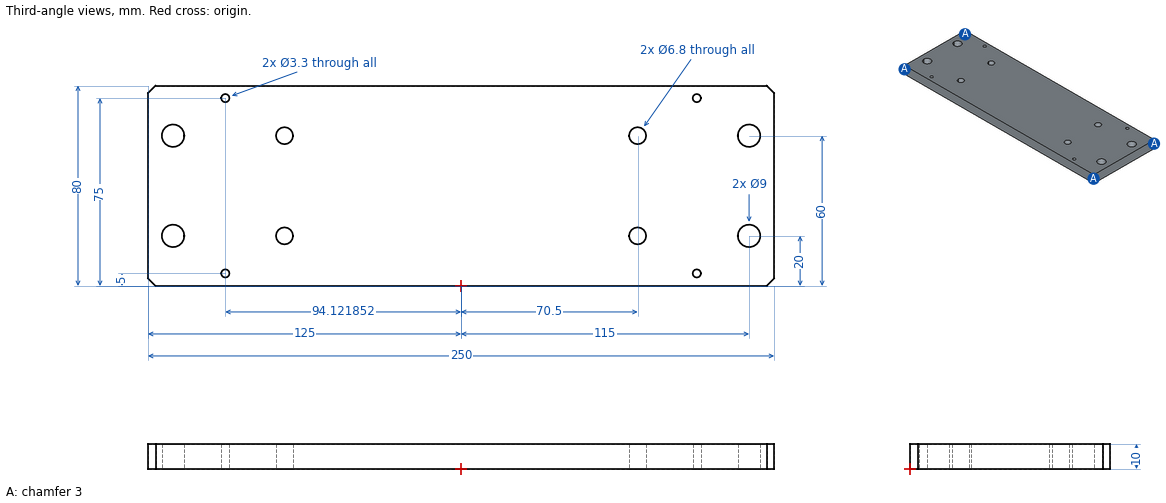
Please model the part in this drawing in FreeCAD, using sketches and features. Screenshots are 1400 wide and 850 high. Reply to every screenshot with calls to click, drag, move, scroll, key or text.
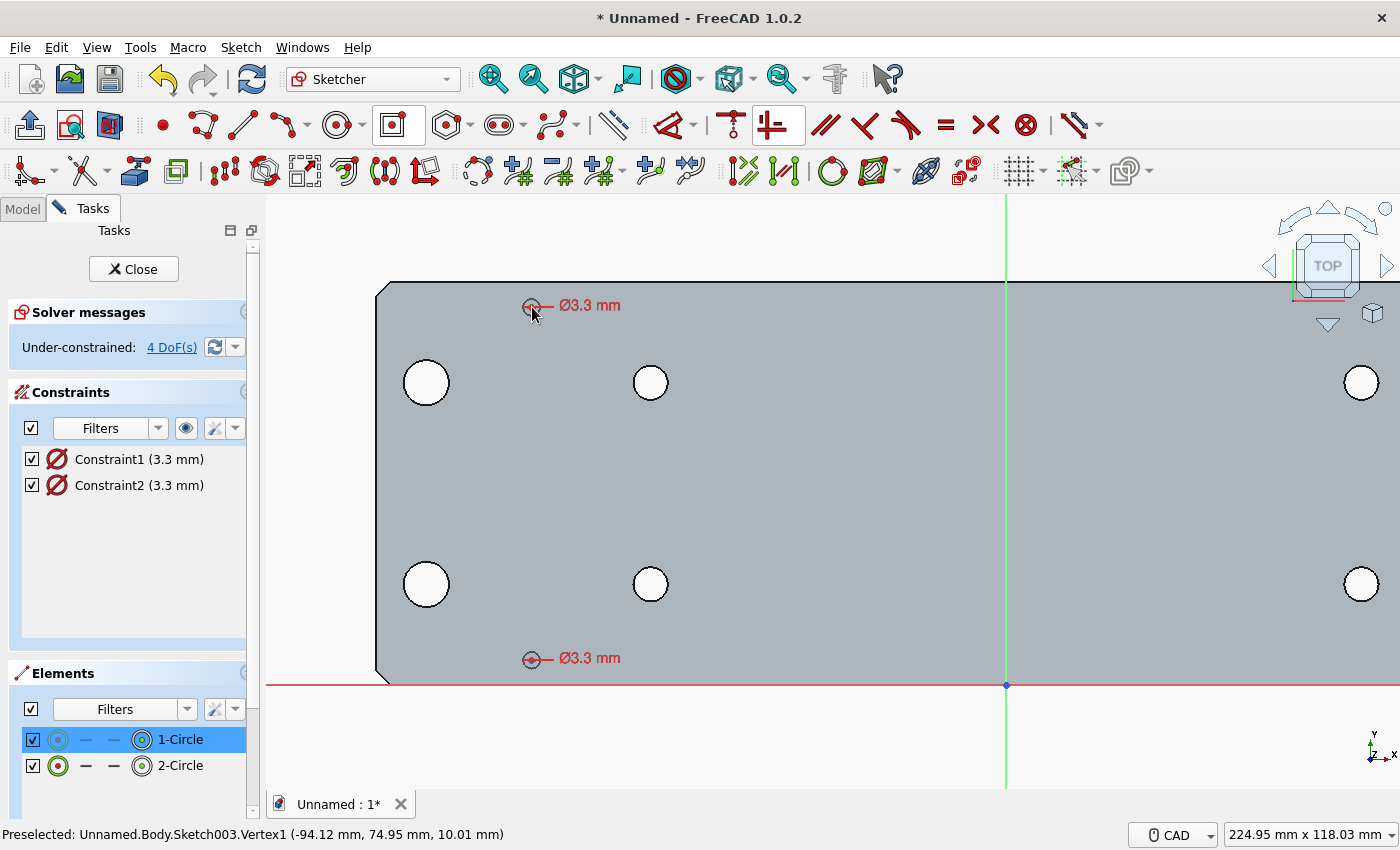
click(532, 660)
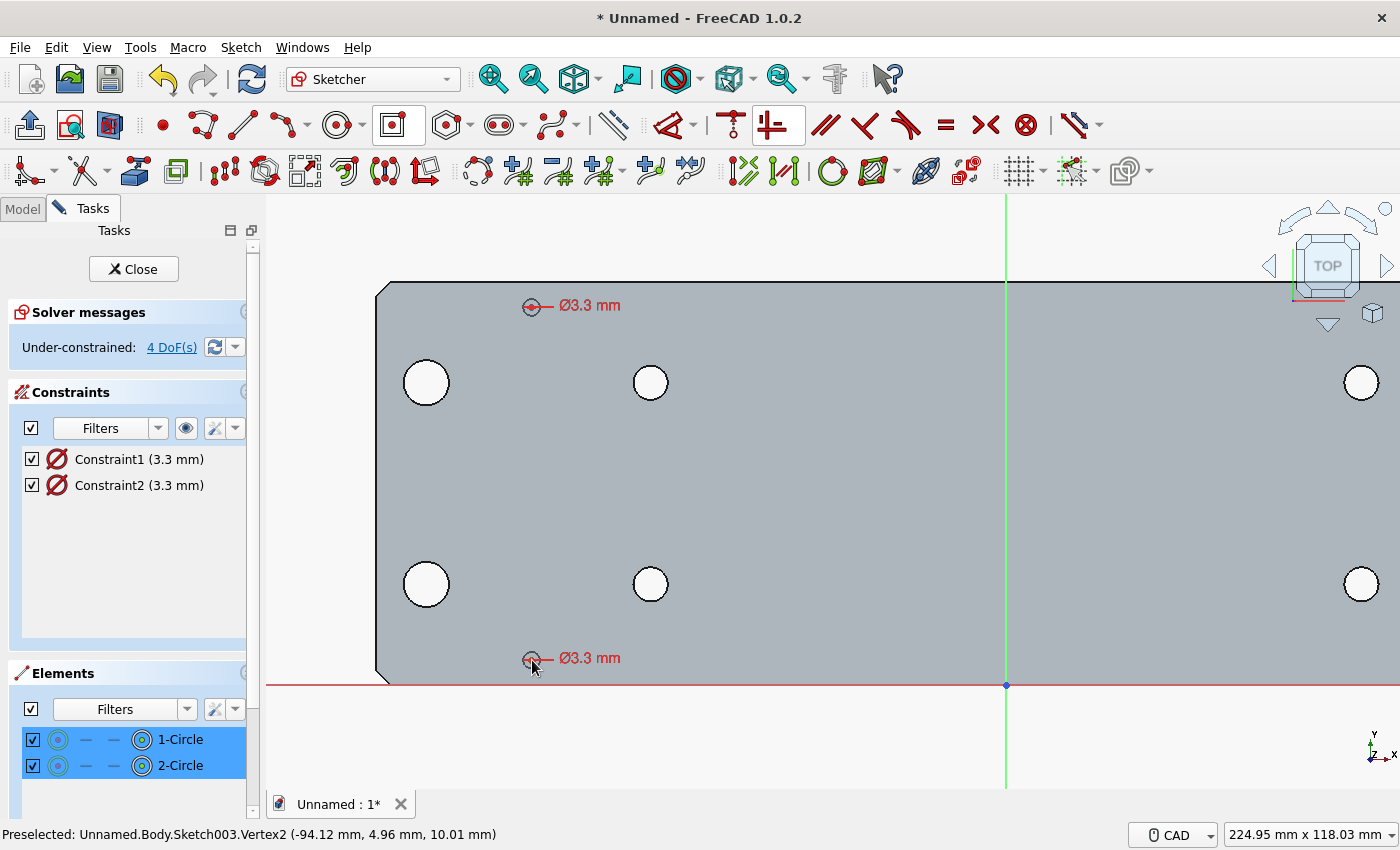
click(800, 126)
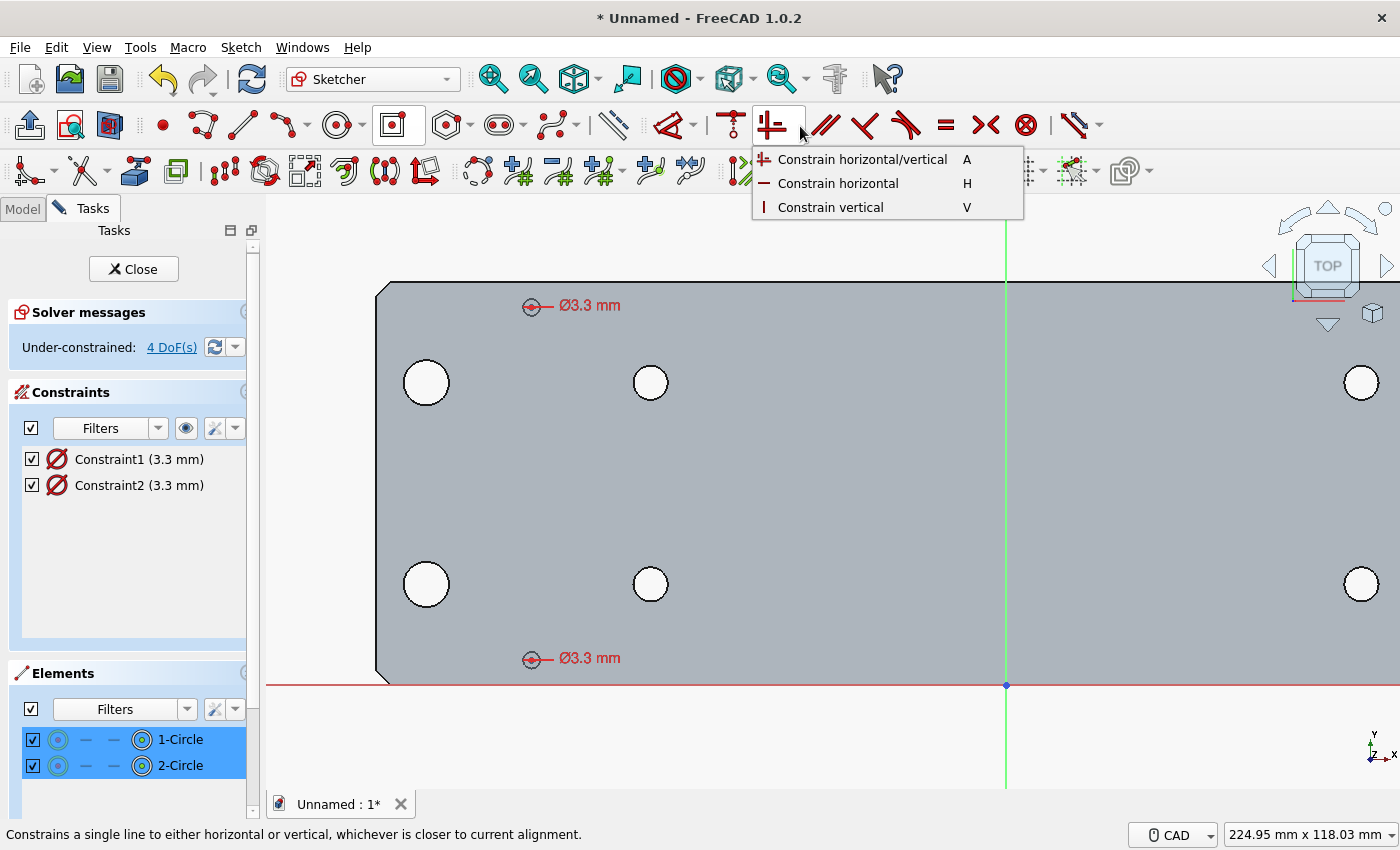
click(888, 207)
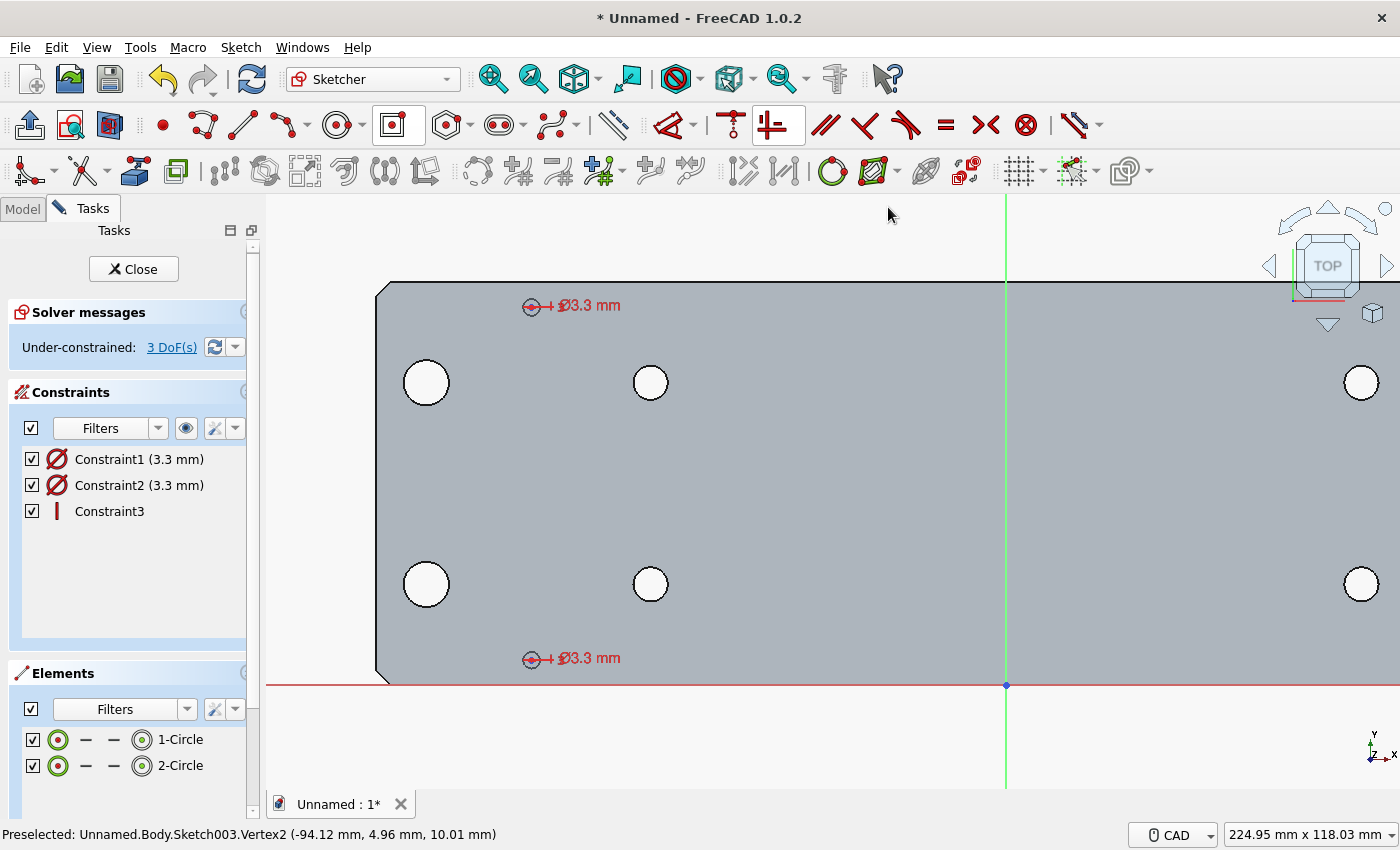
click(668, 126)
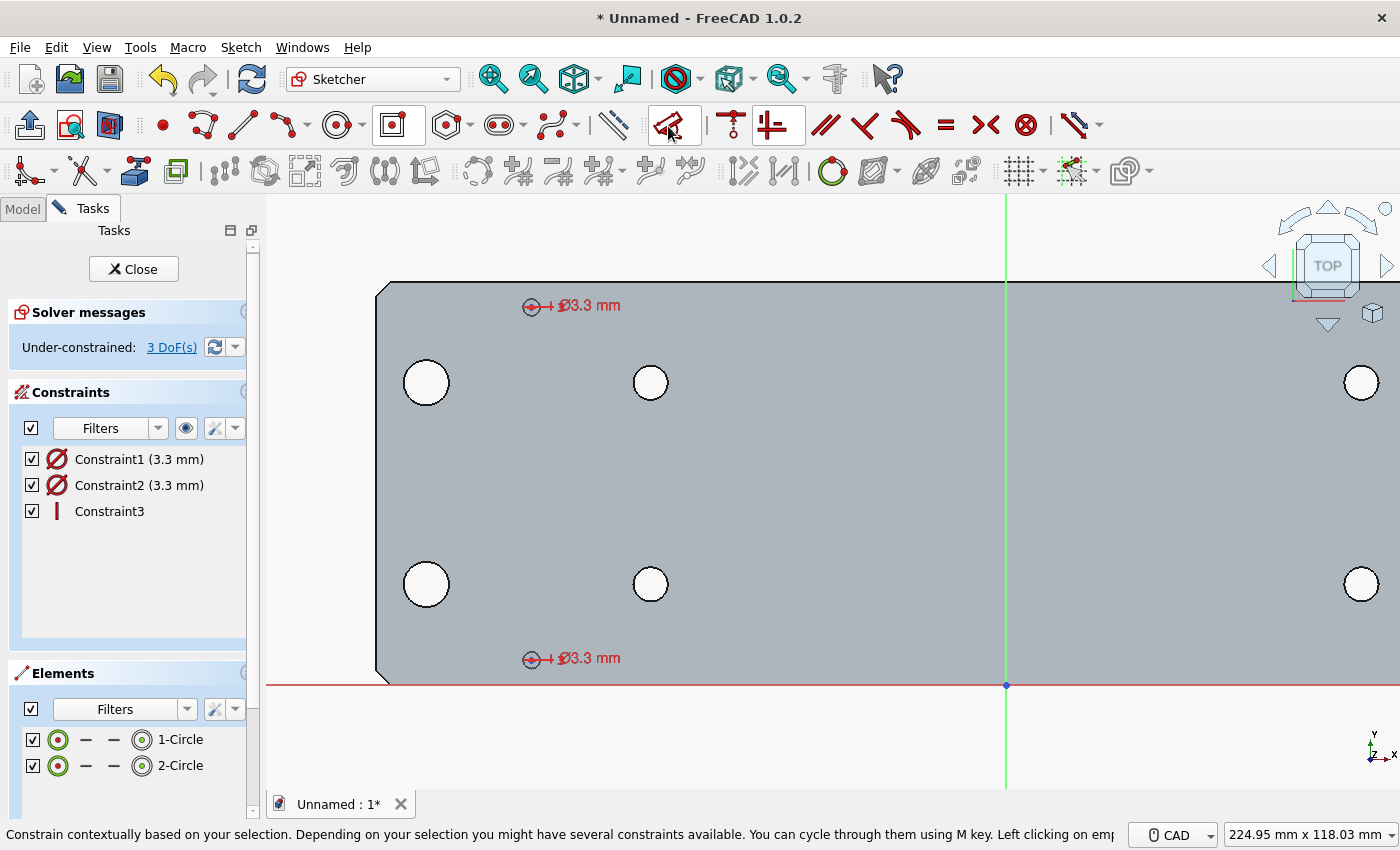
scroll(532, 660, up, 3)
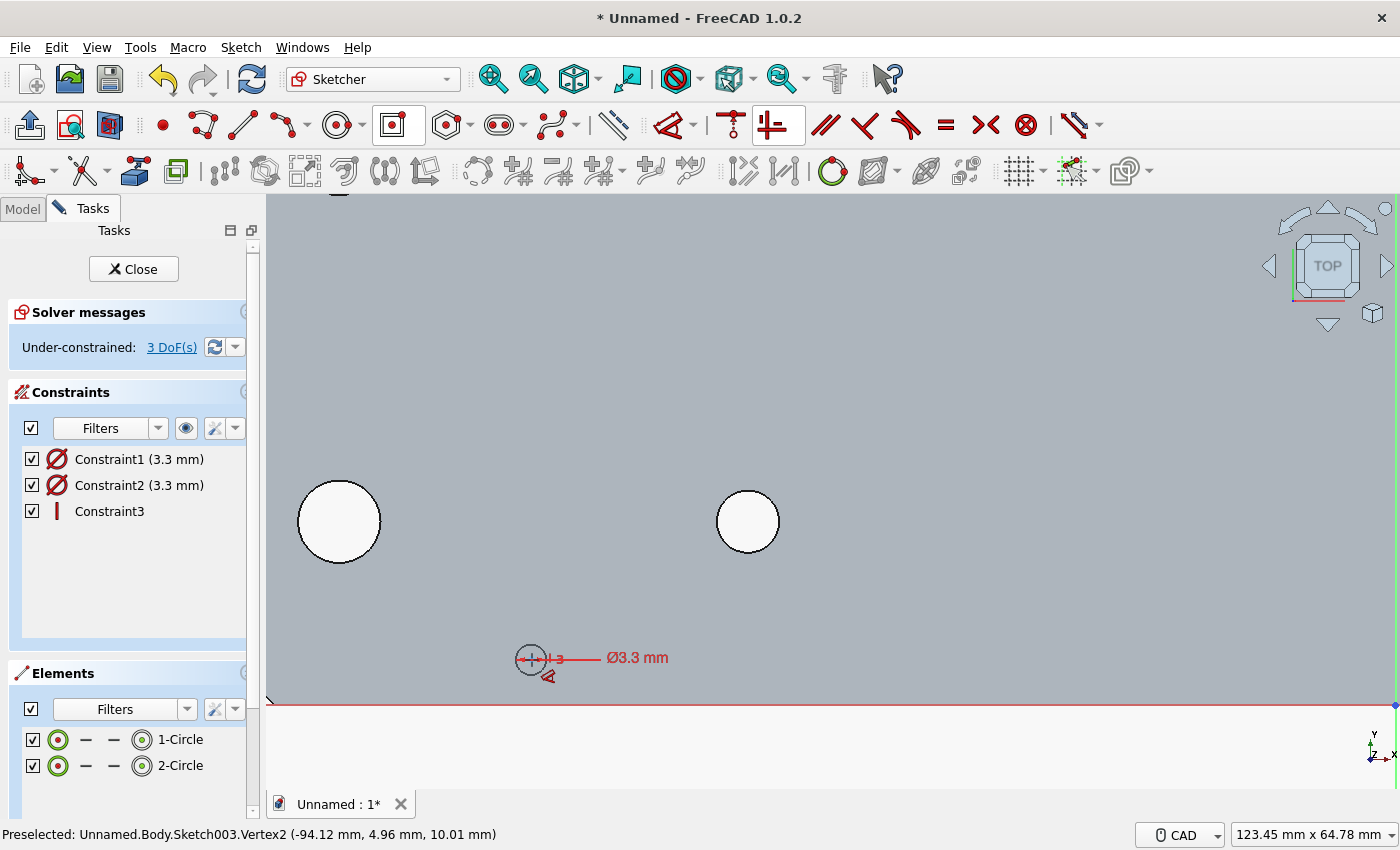
click(531, 660)
click(497, 683)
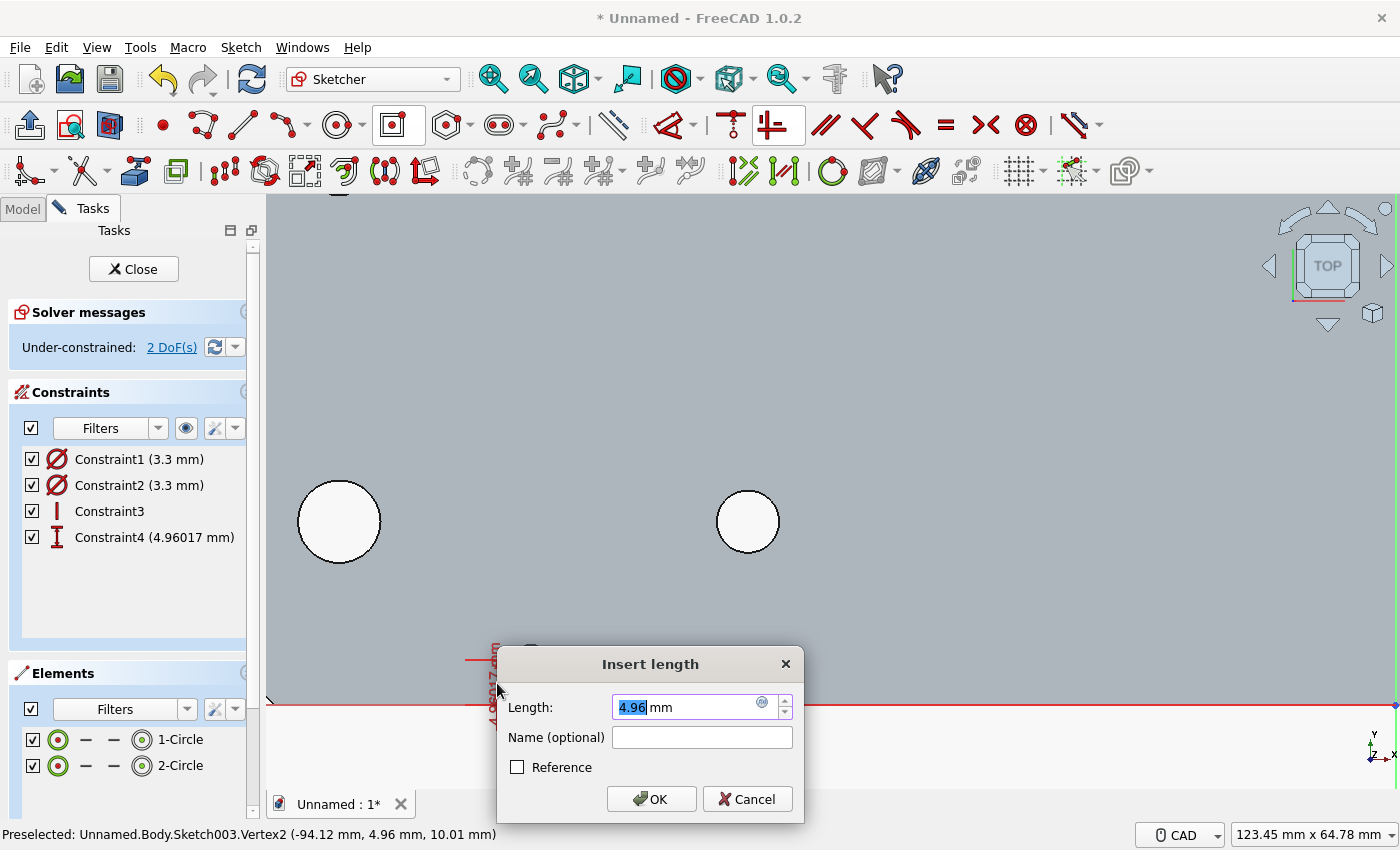
text(5)
key(Return)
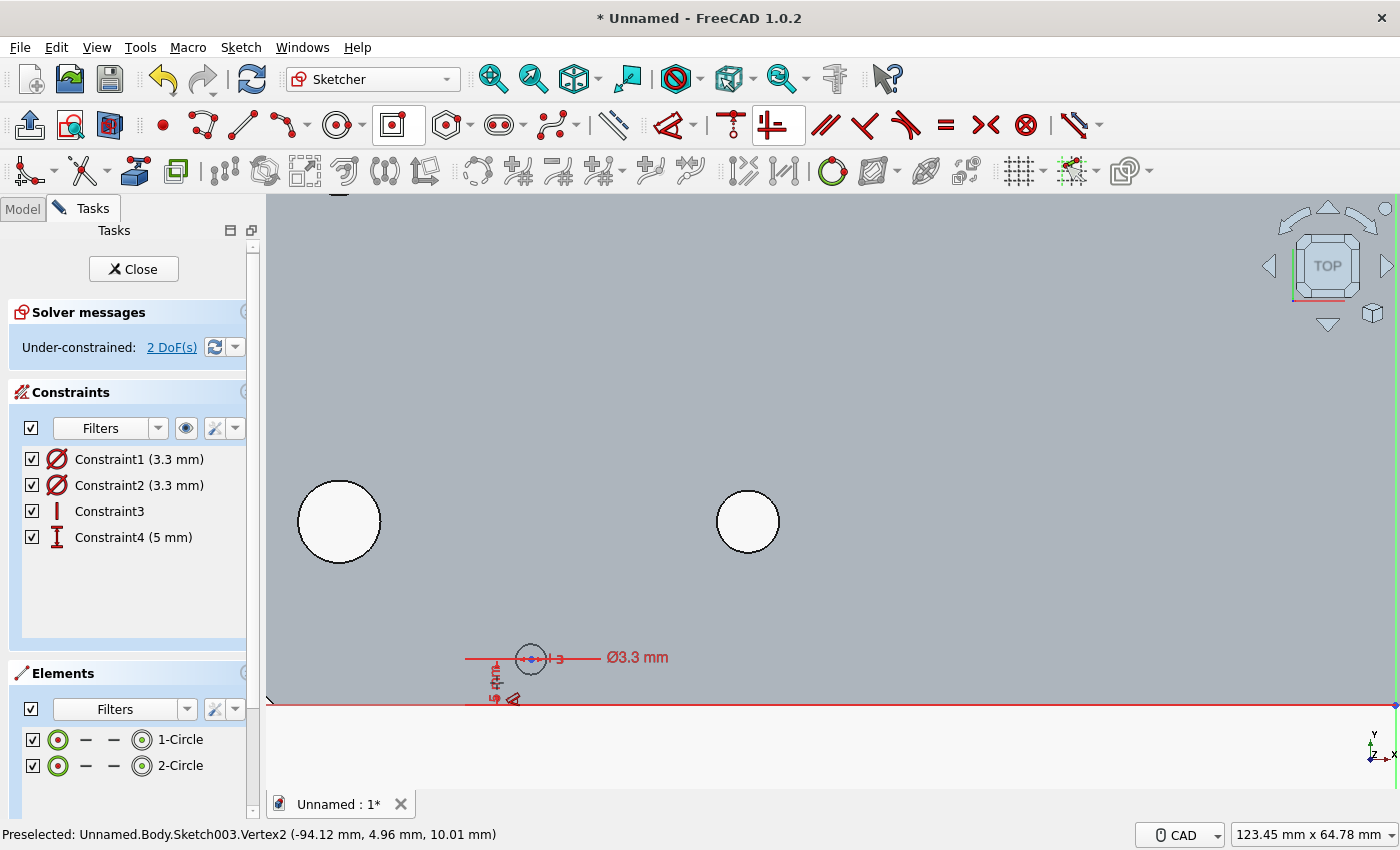
scroll(532, 660, down, 3)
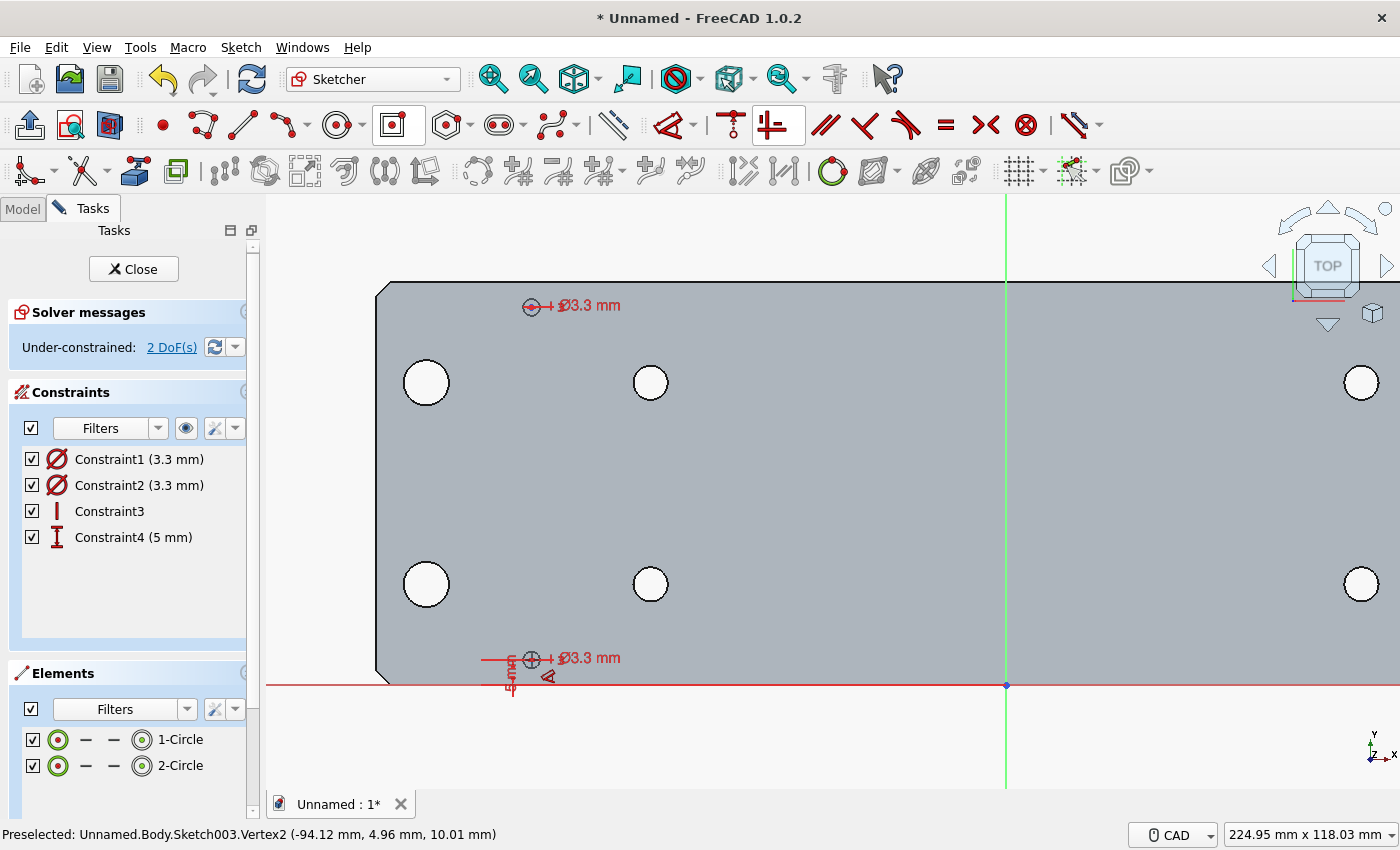
click(532, 307)
click(1040, 496)